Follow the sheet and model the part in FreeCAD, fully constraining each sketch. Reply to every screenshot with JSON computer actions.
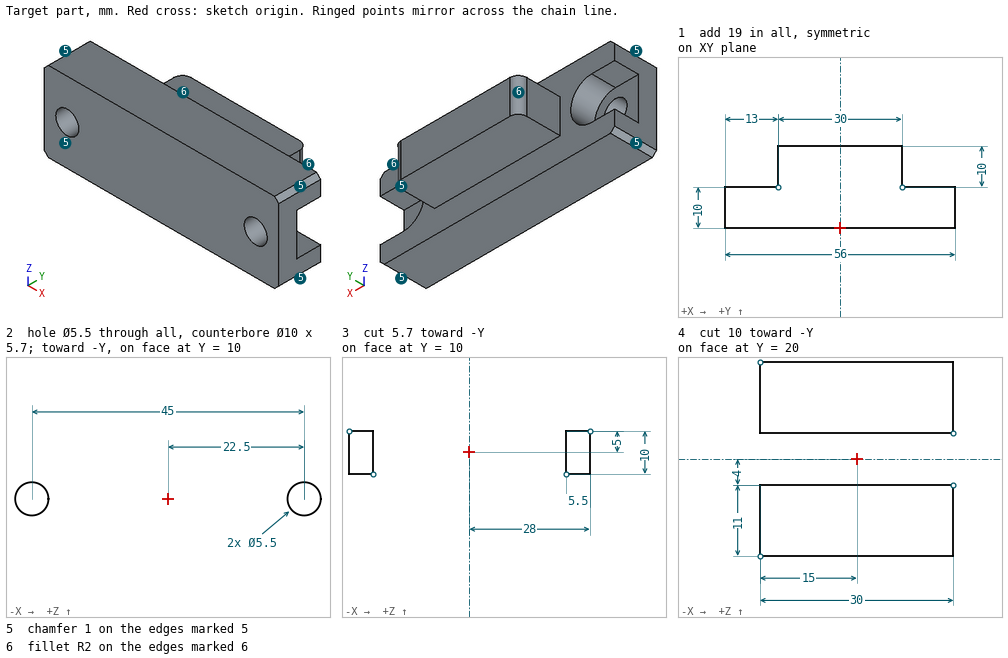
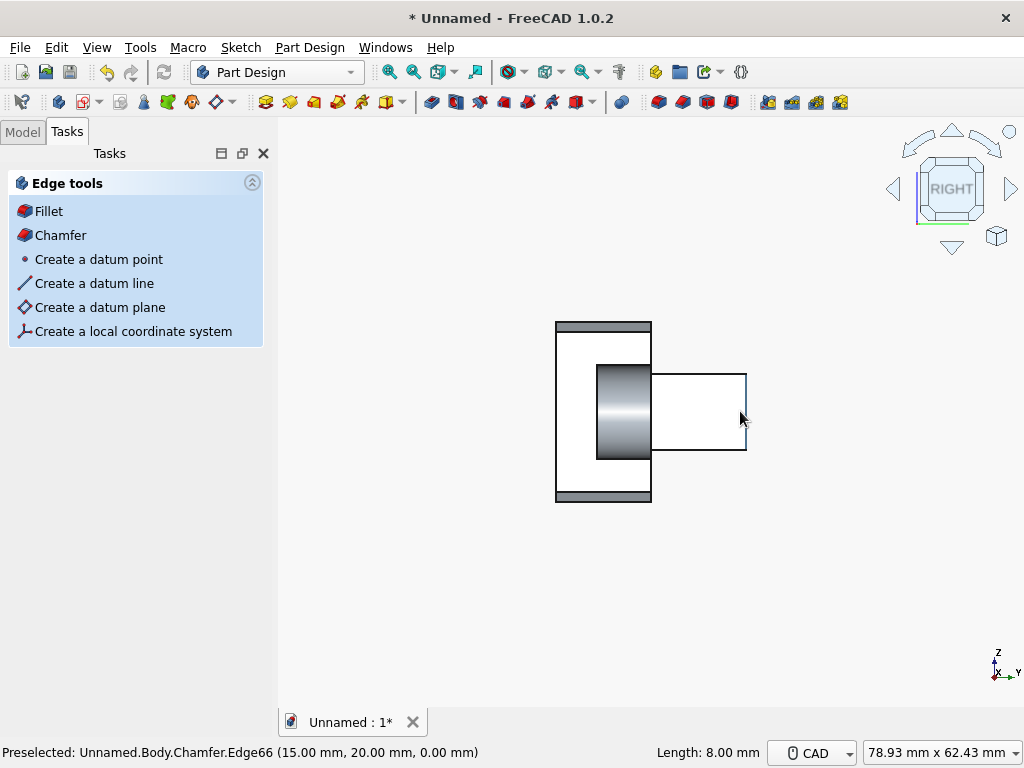
{"action": "key", "text": "5"}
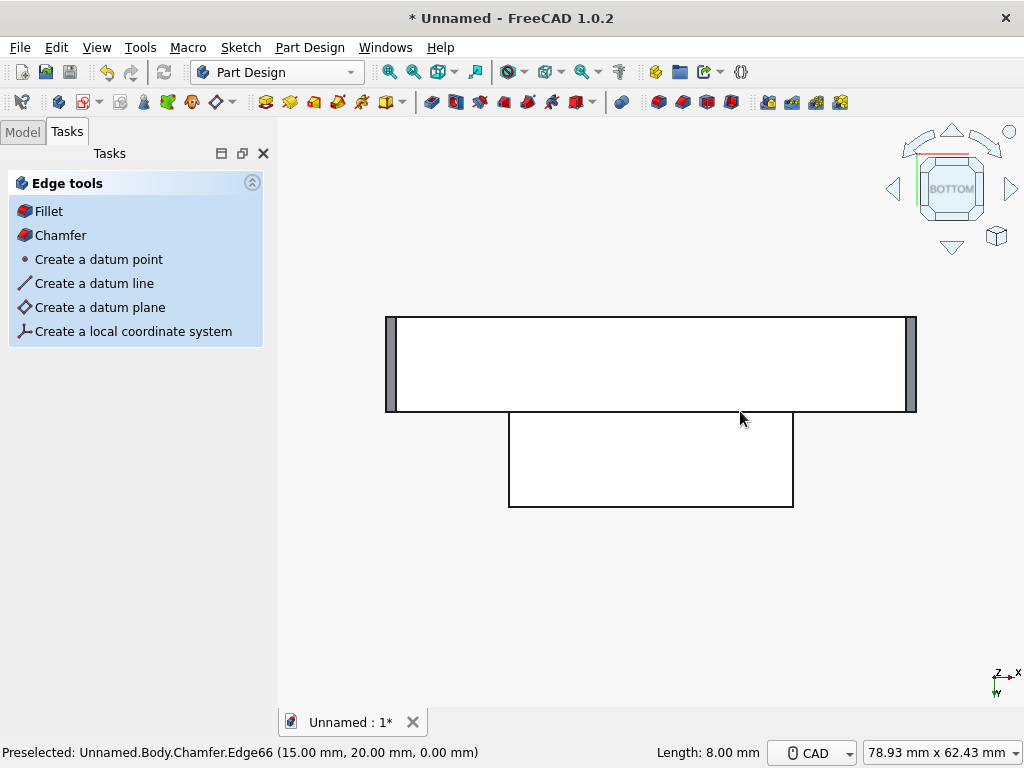
{"action": "key", "text": "4"}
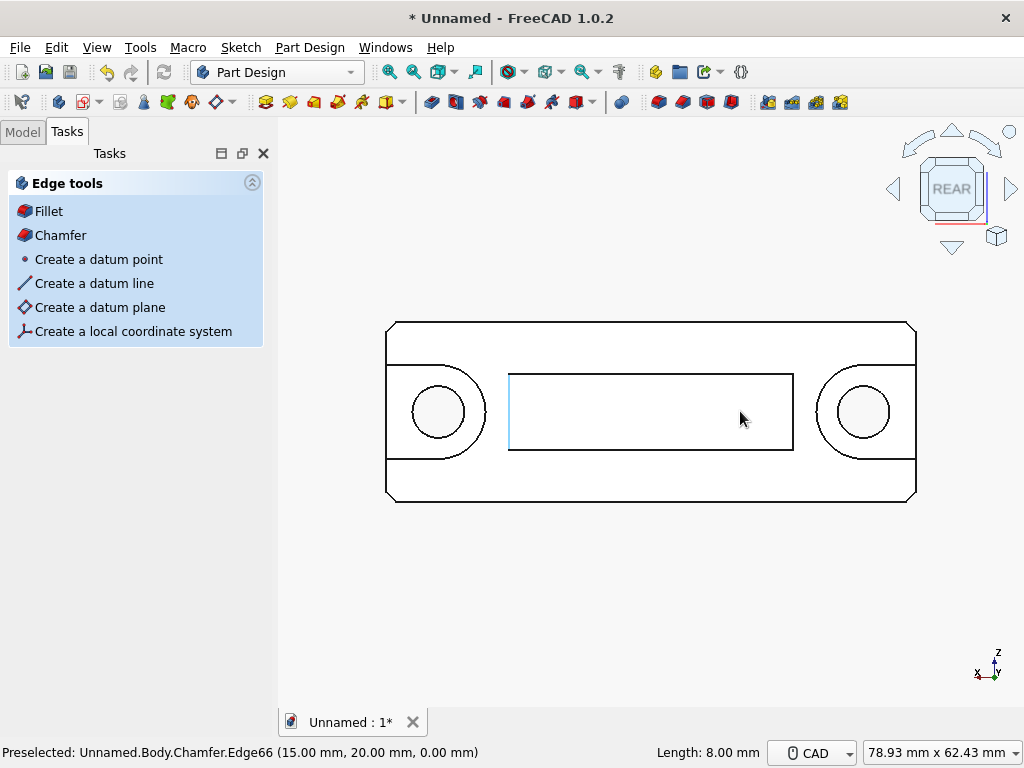
{"action": "left_click", "coordinate": [793, 411], "text": "ctrl"}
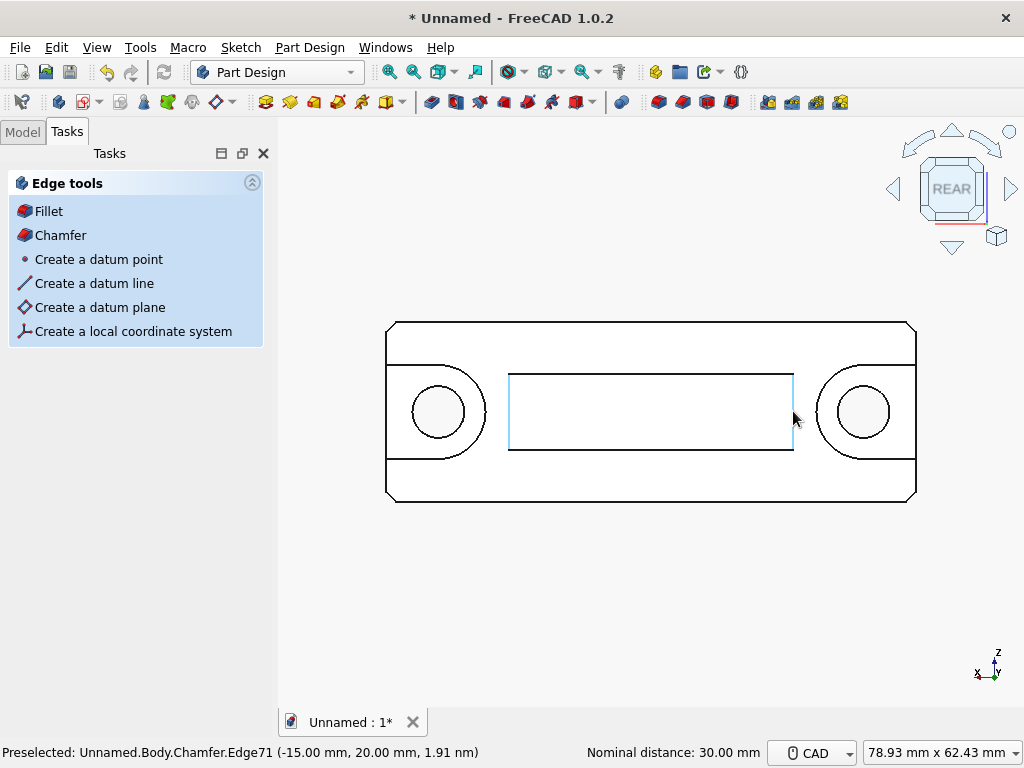
{"action": "left_click", "coordinate": [660, 102]}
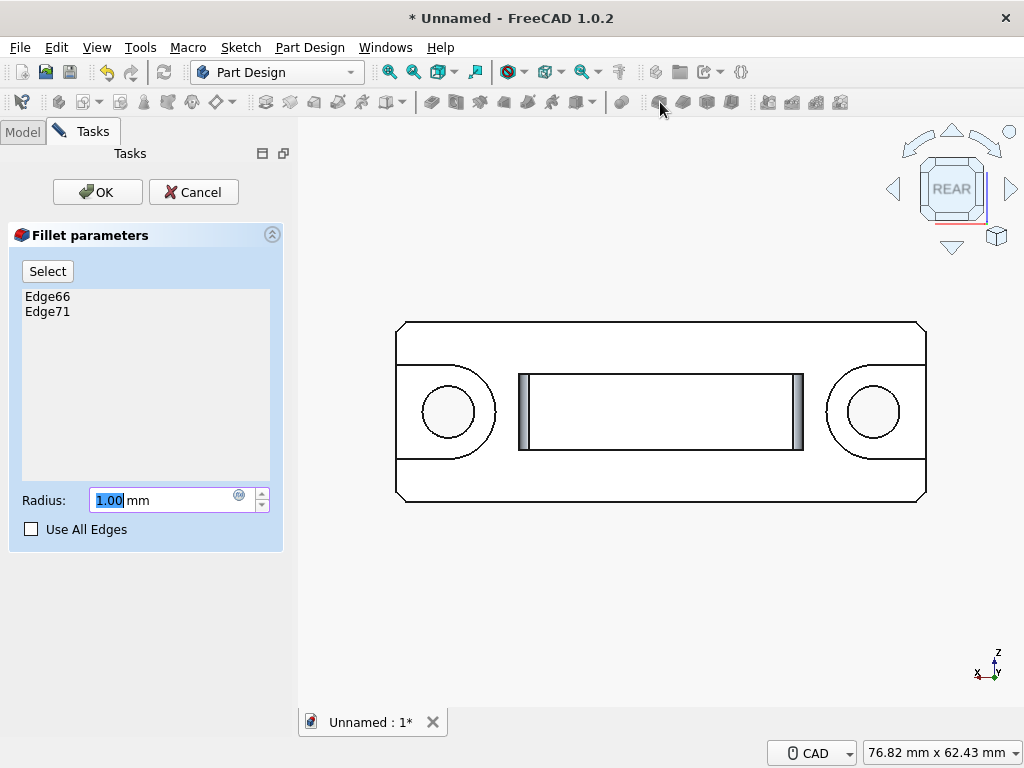
{"action": "type", "text": "2"}
{"action": "key", "text": "Tab"}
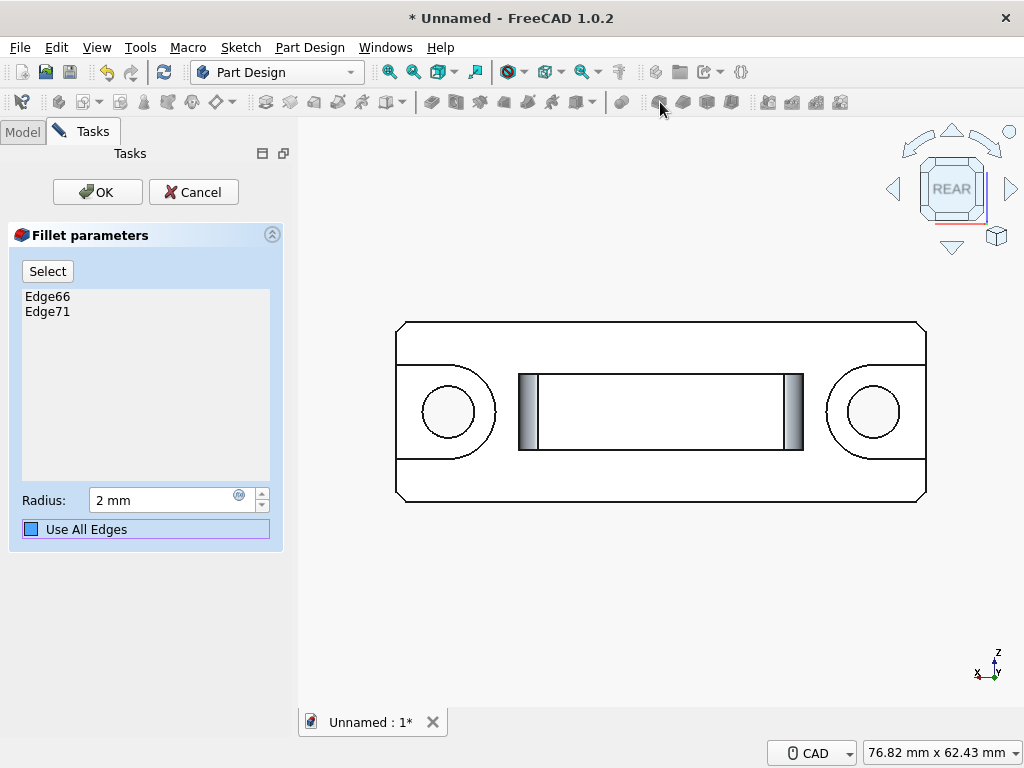
{"action": "left_click", "coordinate": [98, 192]}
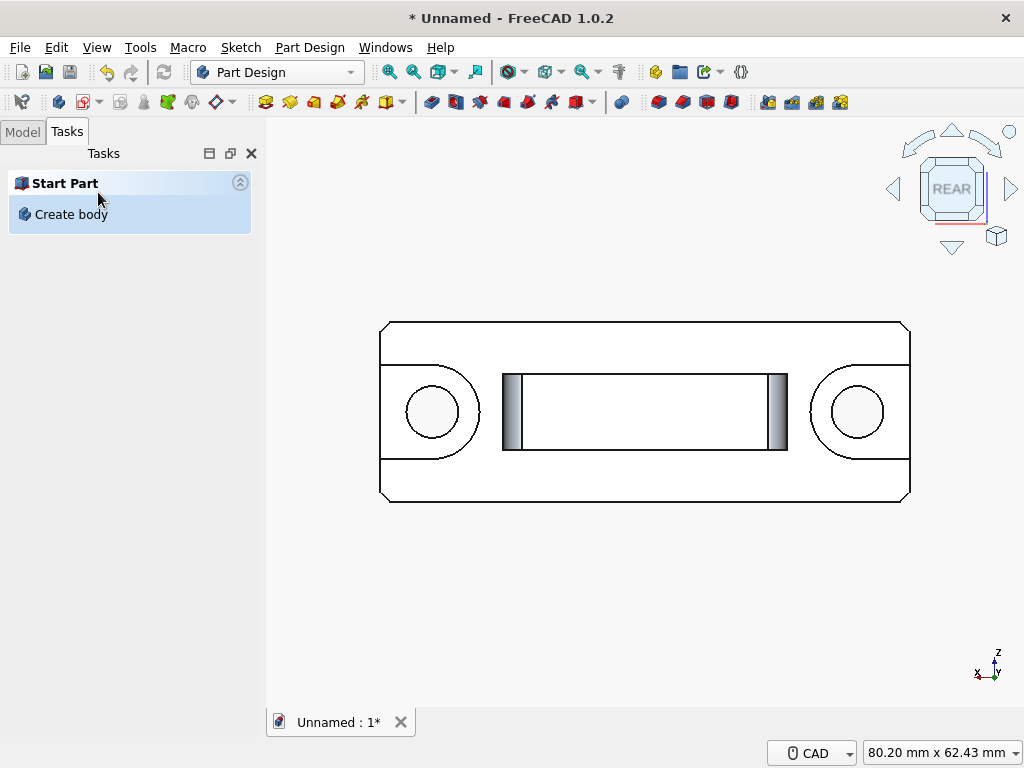
{"action": "key", "text": "0"}